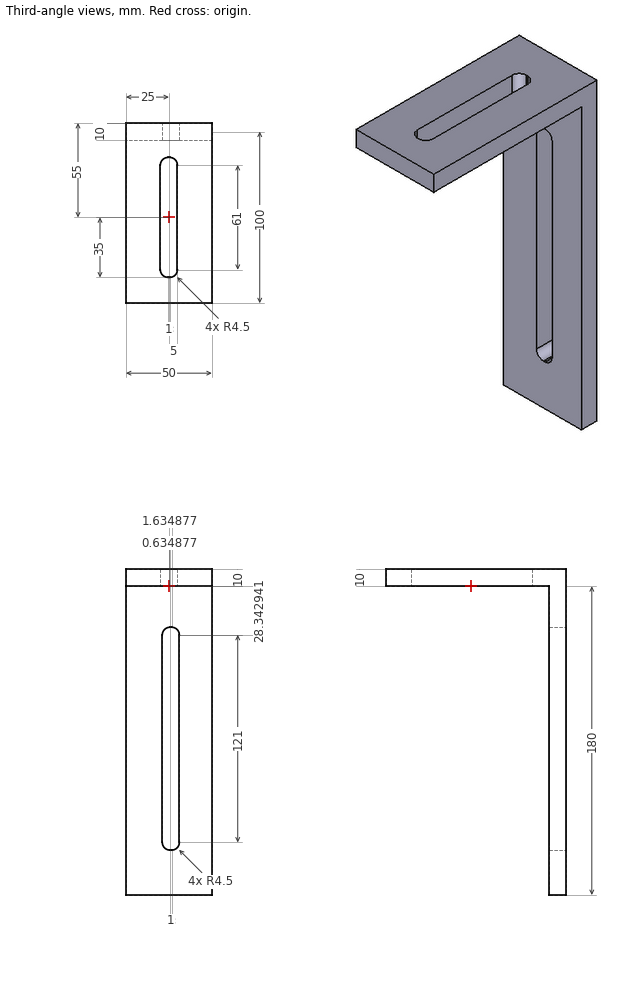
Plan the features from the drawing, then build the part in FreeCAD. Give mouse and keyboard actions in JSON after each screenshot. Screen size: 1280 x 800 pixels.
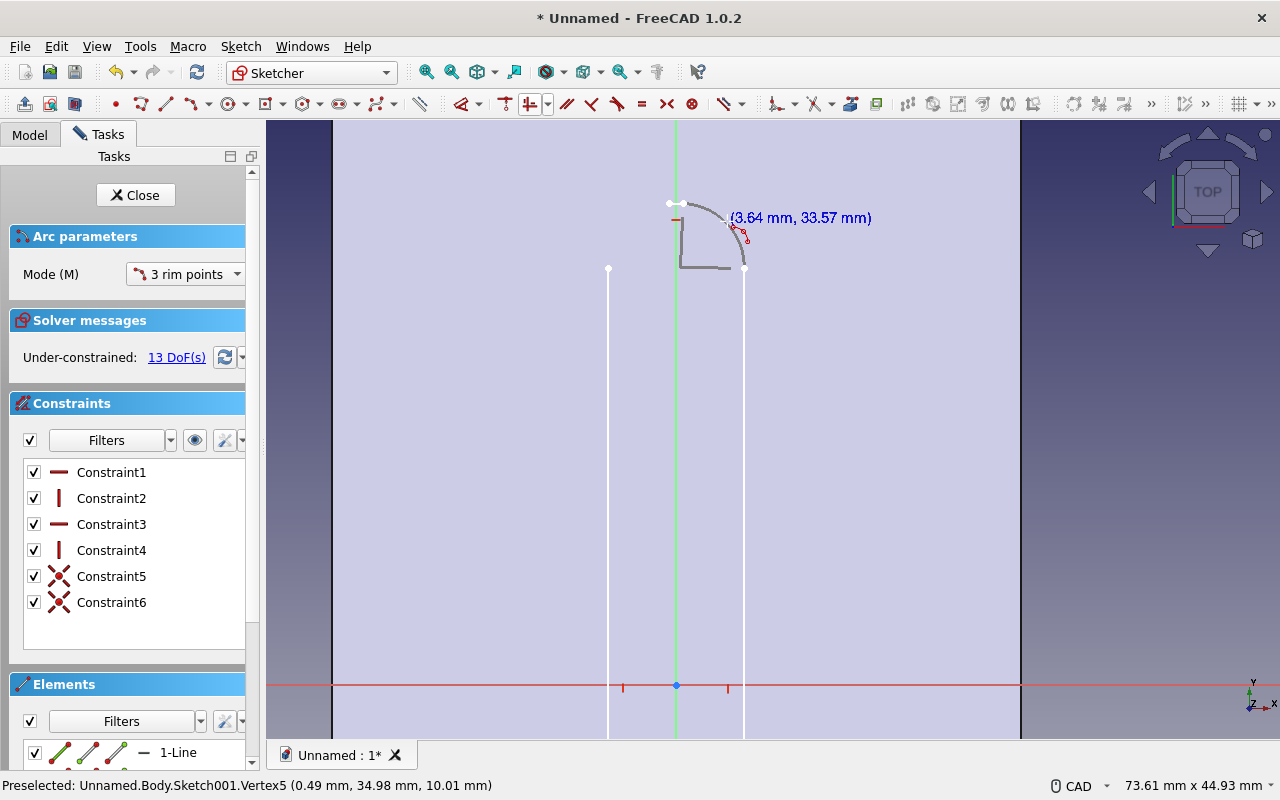
{"action": "left_click", "coordinate": [727, 221]}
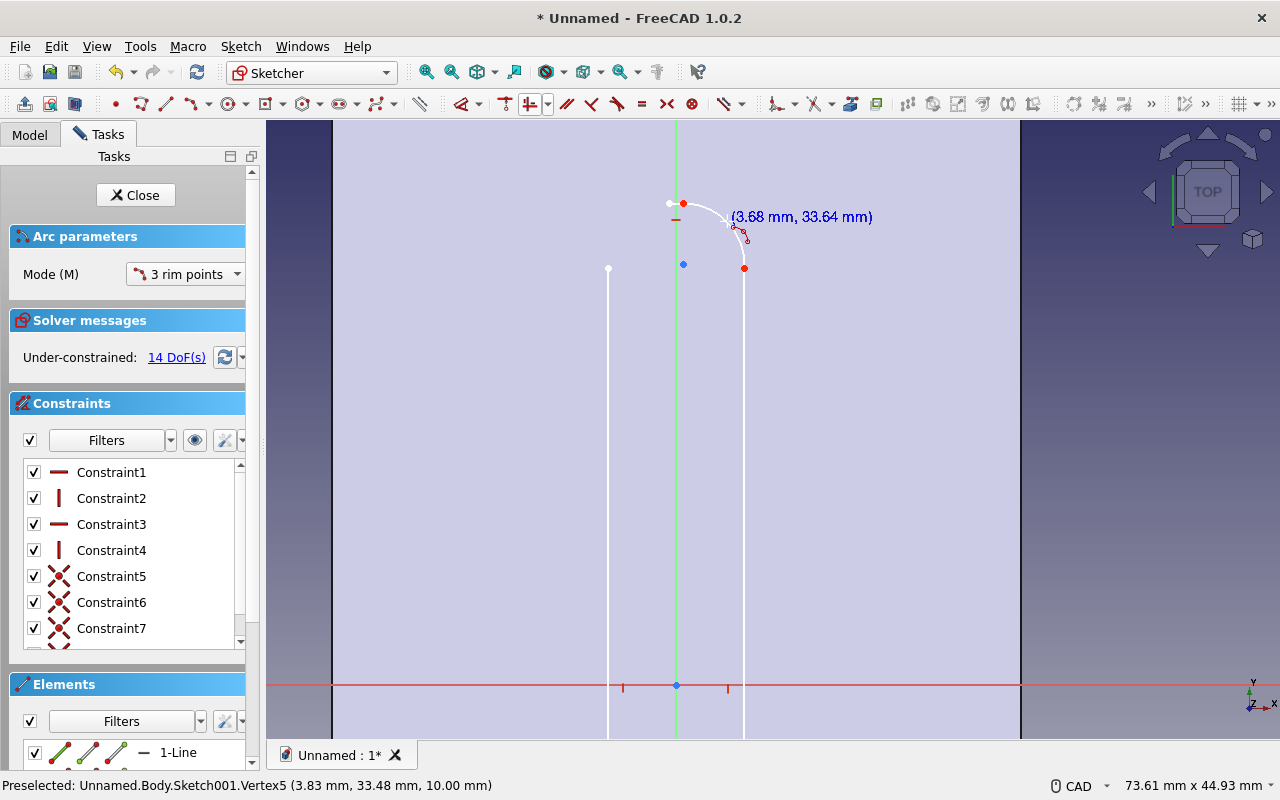
{"action": "scroll", "coordinate": [669, 203], "scroll_direction": "up", "scroll_amount": 5}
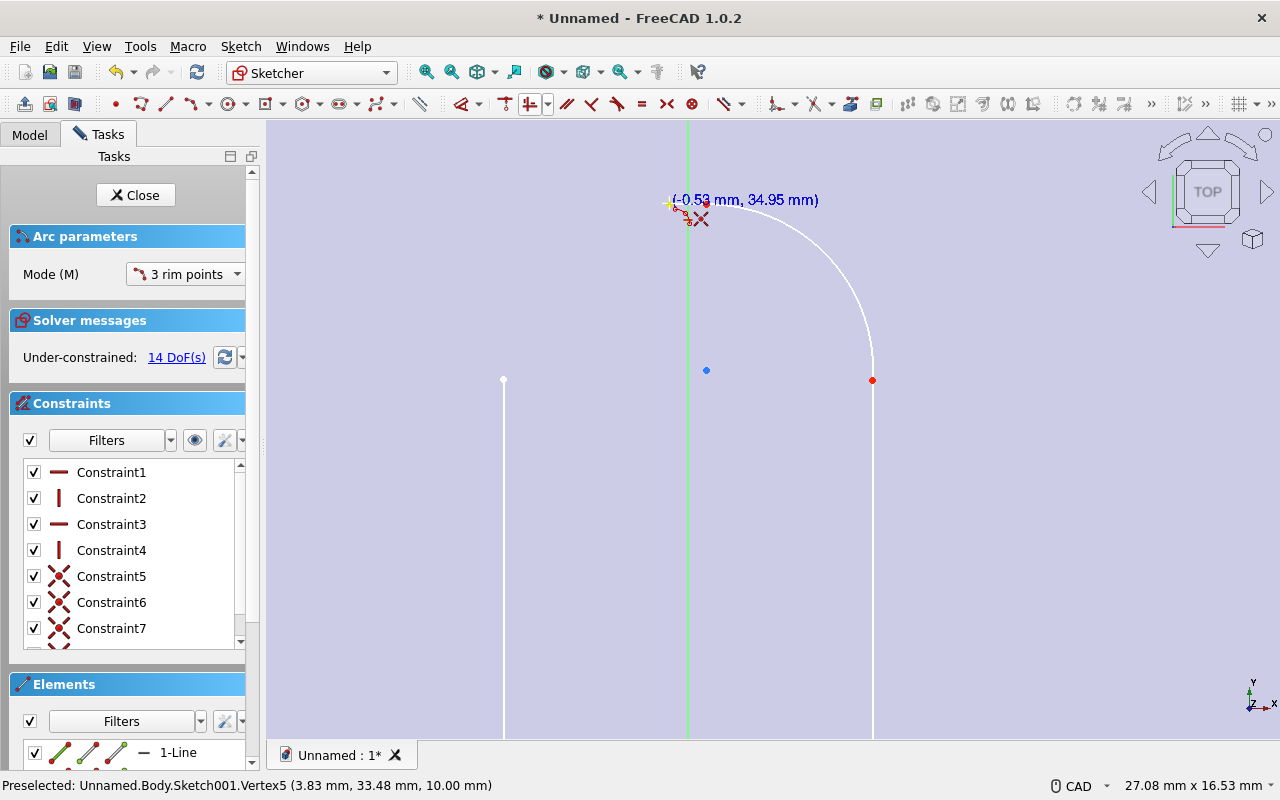
{"action": "left_click", "coordinate": [670, 204]}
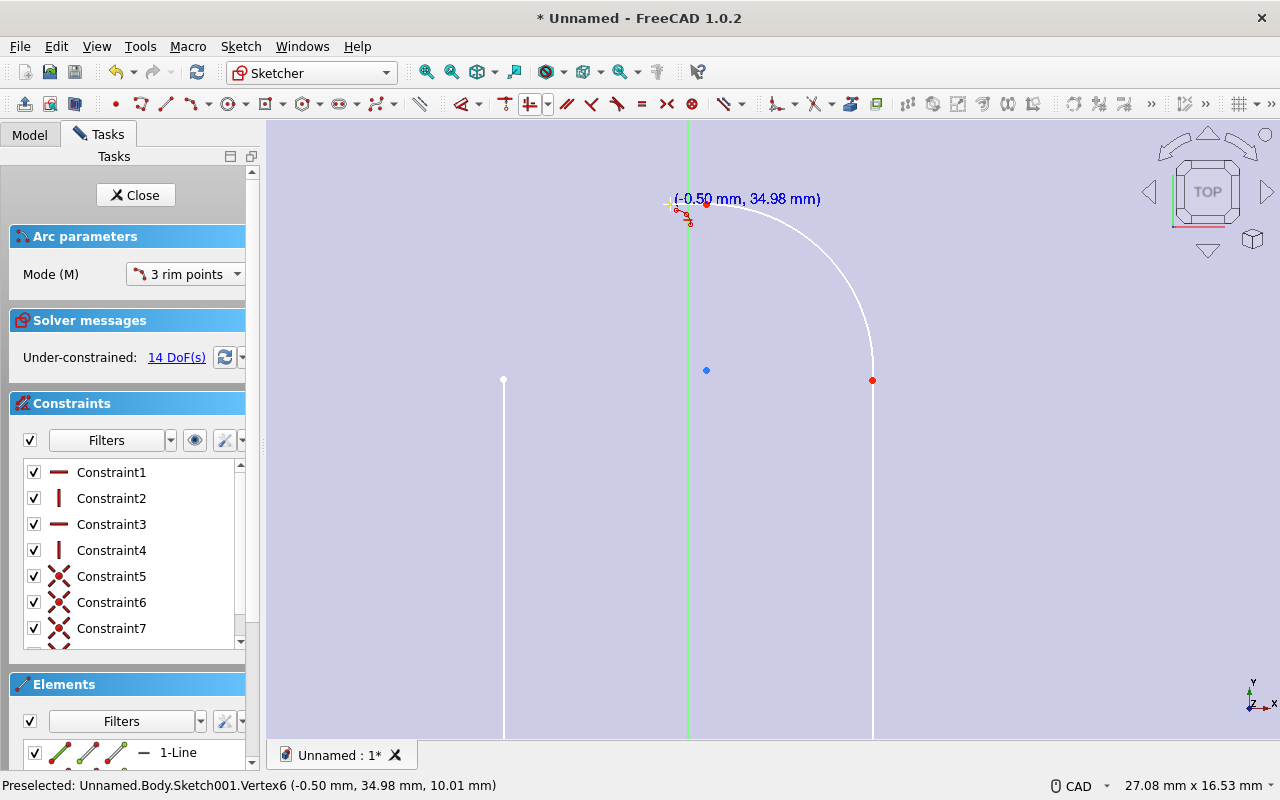
{"action": "scroll", "coordinate": [708, 215], "scroll_direction": "down", "scroll_amount": 9}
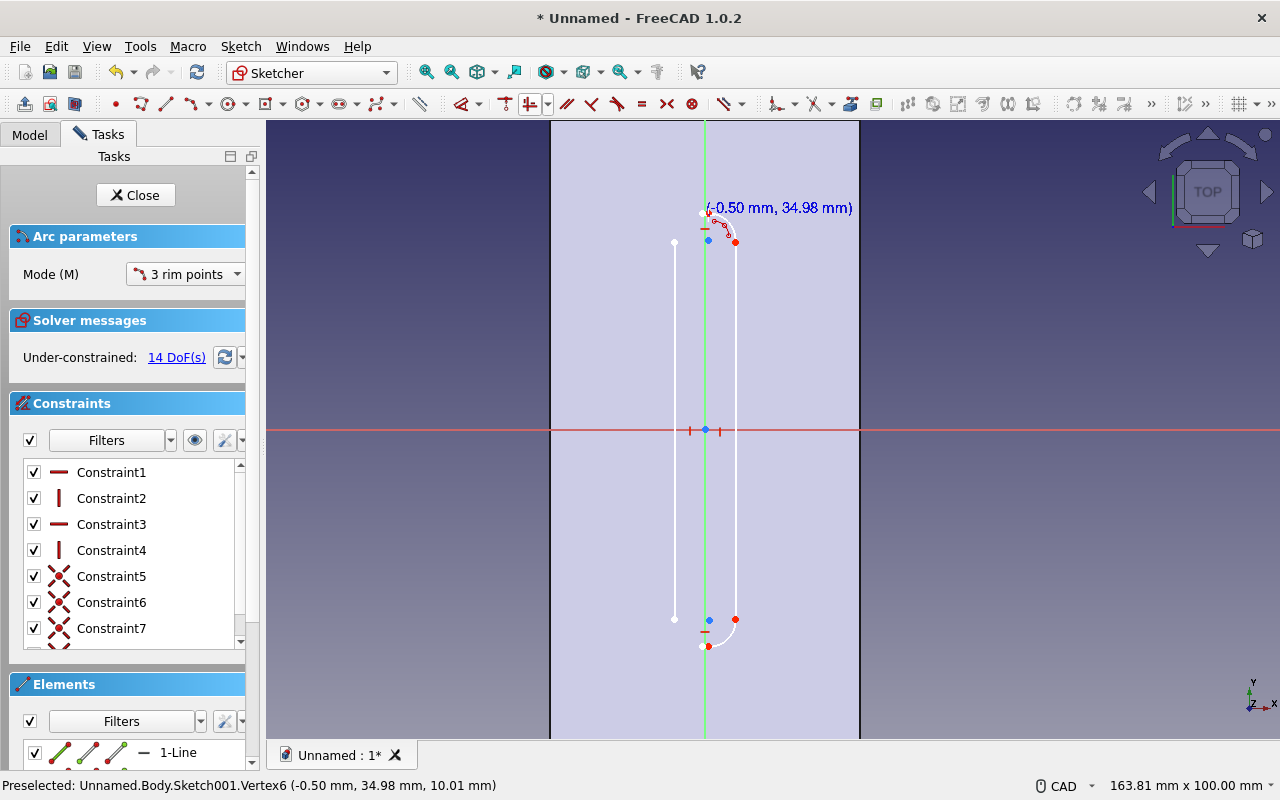
{"action": "left_click", "coordinate": [675, 242]}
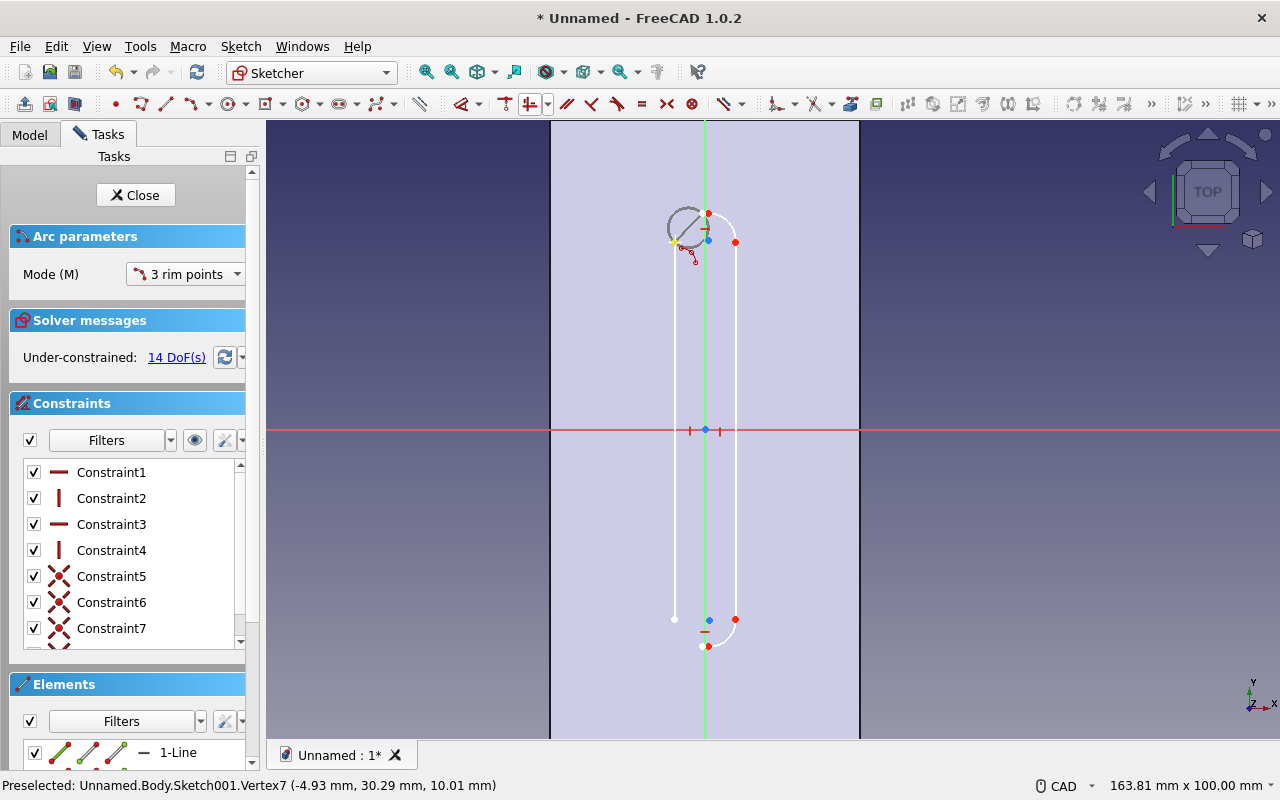
{"action": "scroll", "coordinate": [682, 221], "scroll_direction": "up", "scroll_amount": 4}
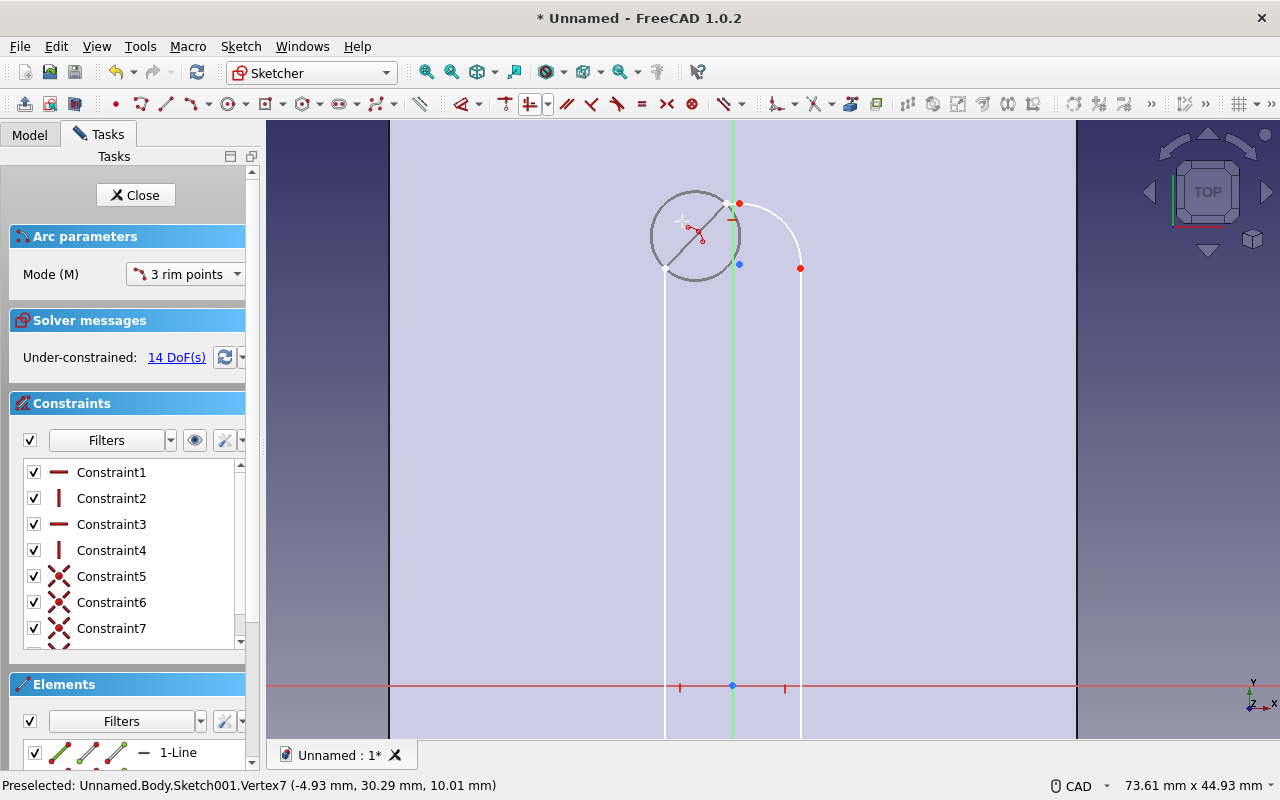
{"action": "left_click", "coordinate": [682, 222]}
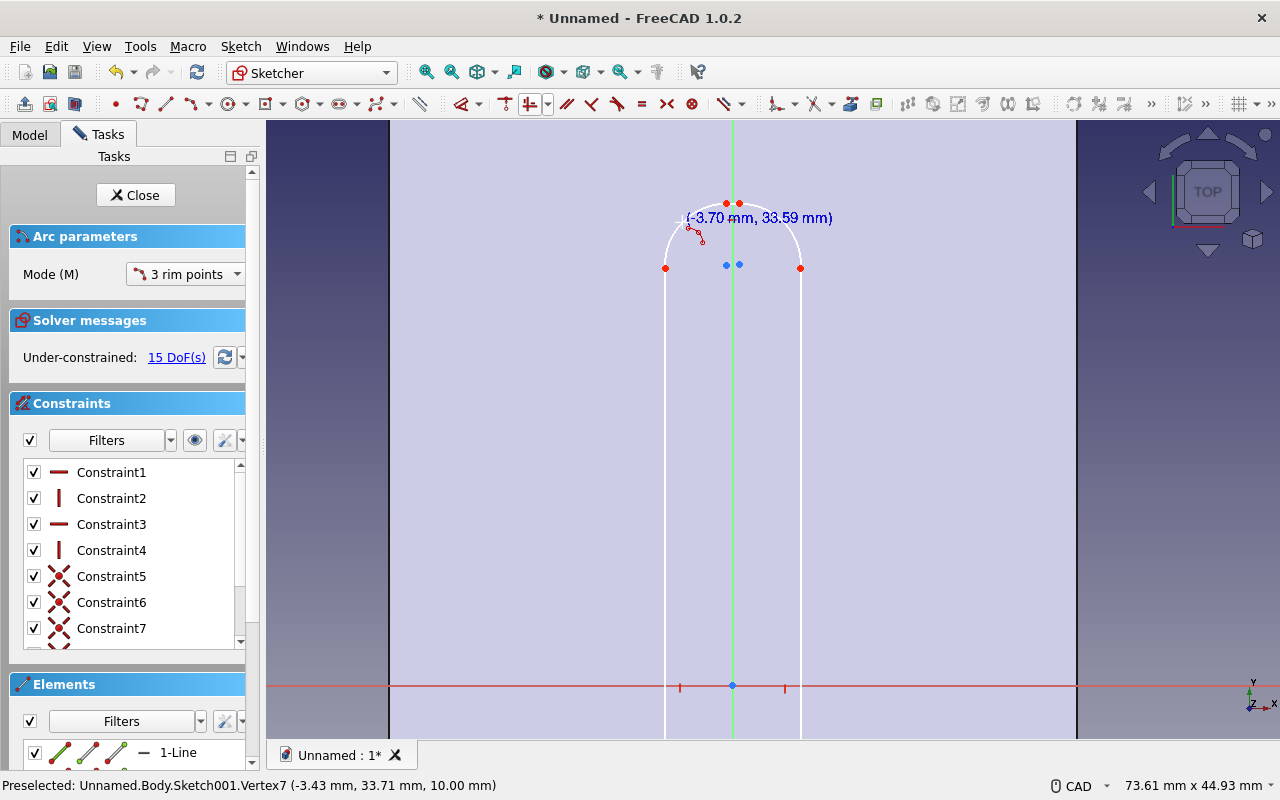
{"action": "scroll", "coordinate": [681, 220], "scroll_direction": "down", "scroll_amount": 4}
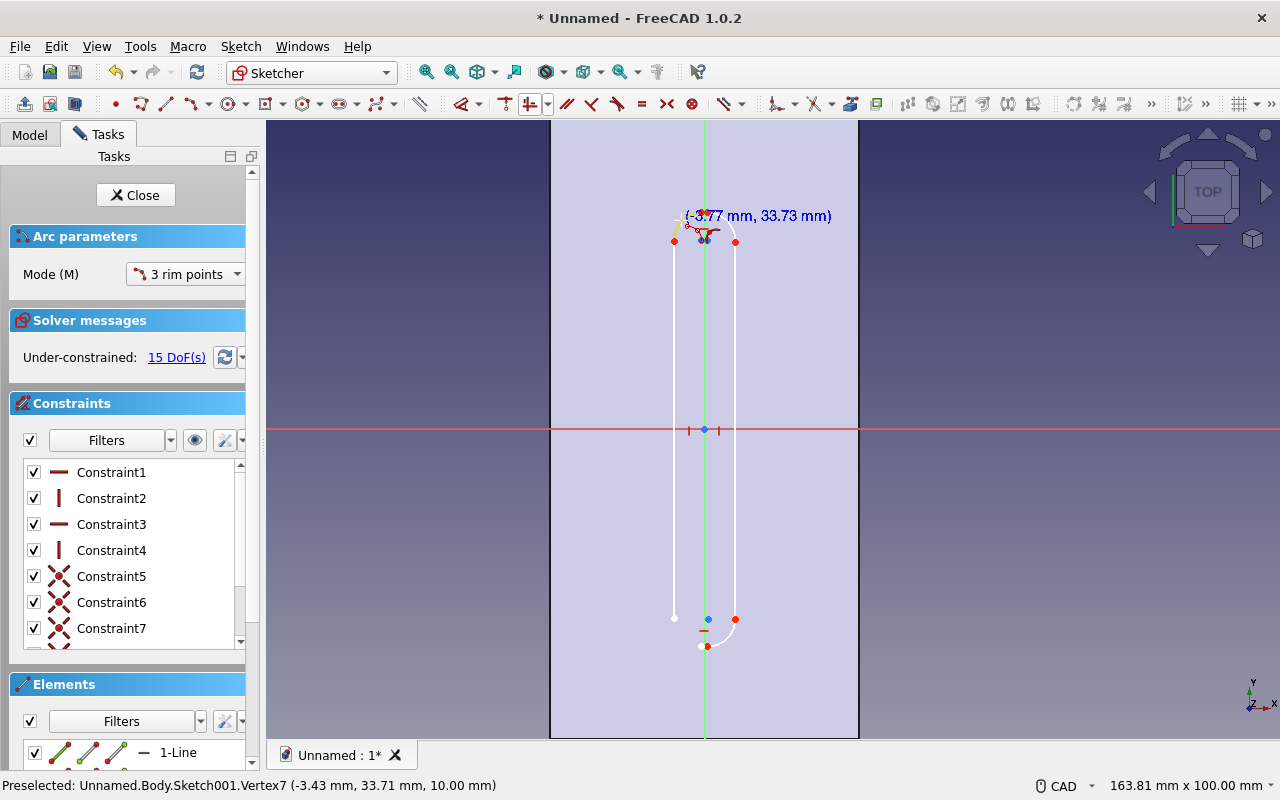
{"action": "left_click", "coordinate": [674, 619]}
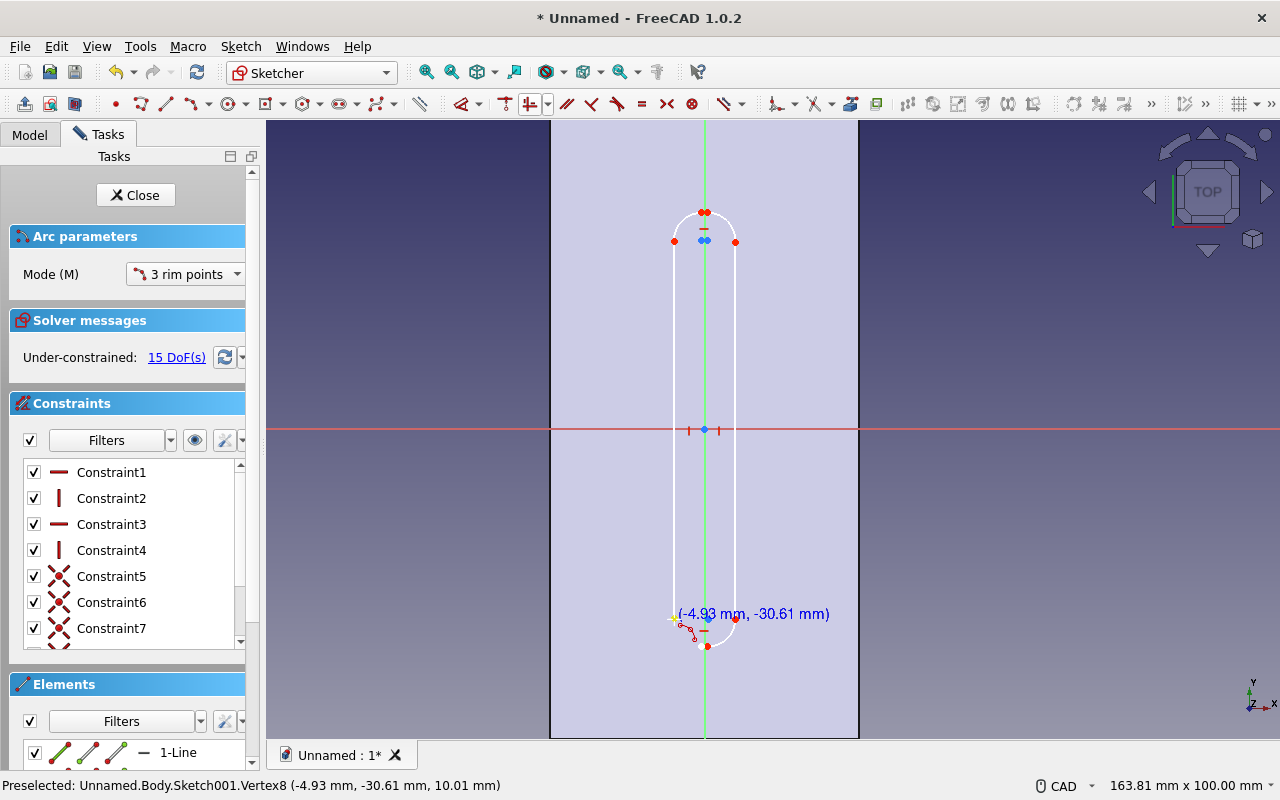
{"action": "scroll", "coordinate": [701, 646], "scroll_direction": "up", "scroll_amount": 9}